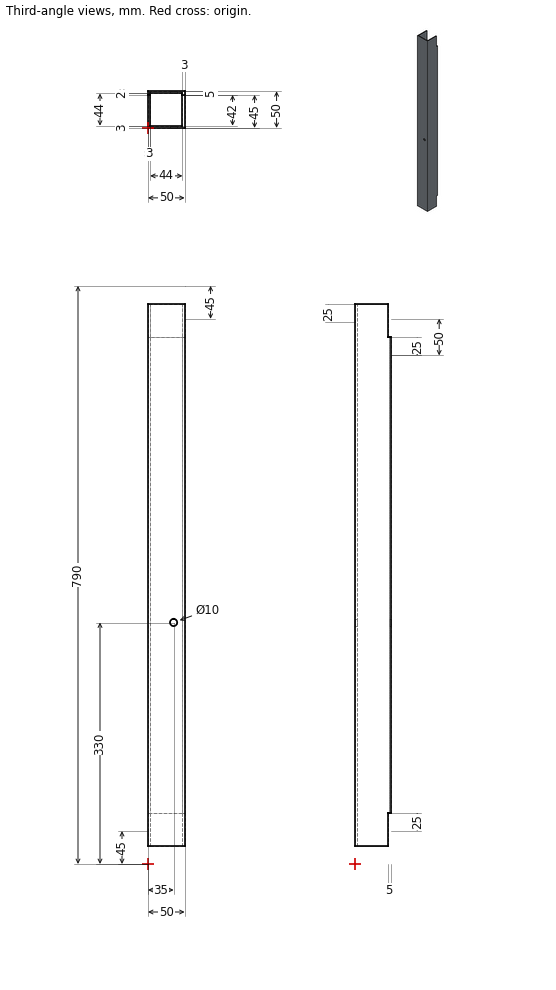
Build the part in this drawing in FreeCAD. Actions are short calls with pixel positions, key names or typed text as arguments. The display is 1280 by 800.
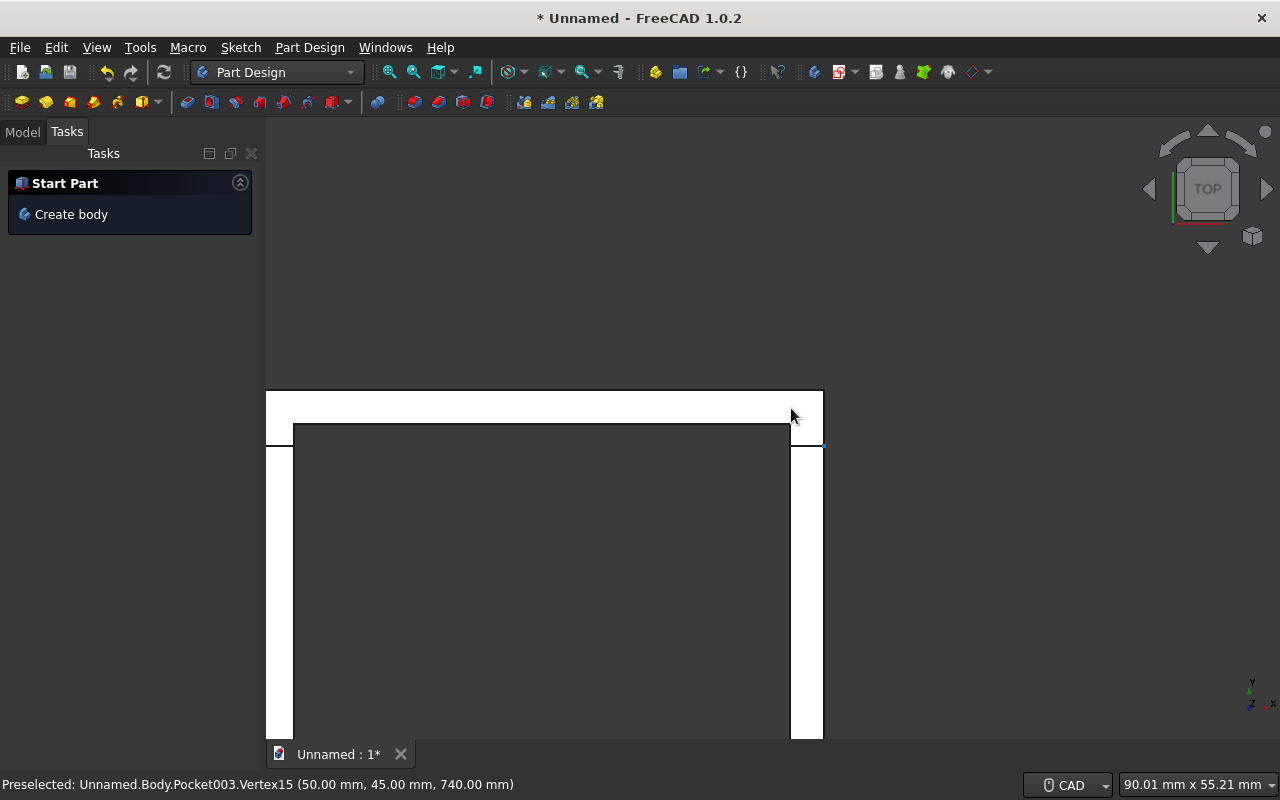
click(784, 409)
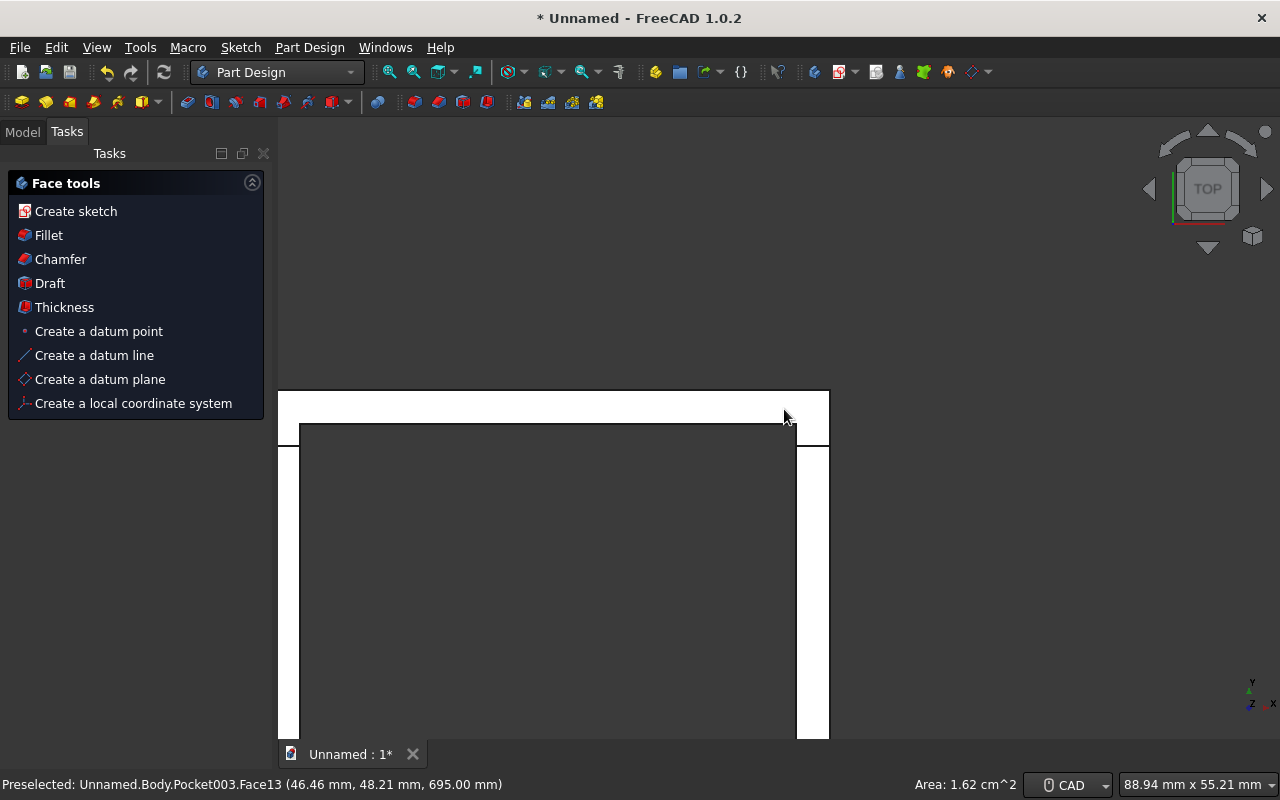
click(840, 72)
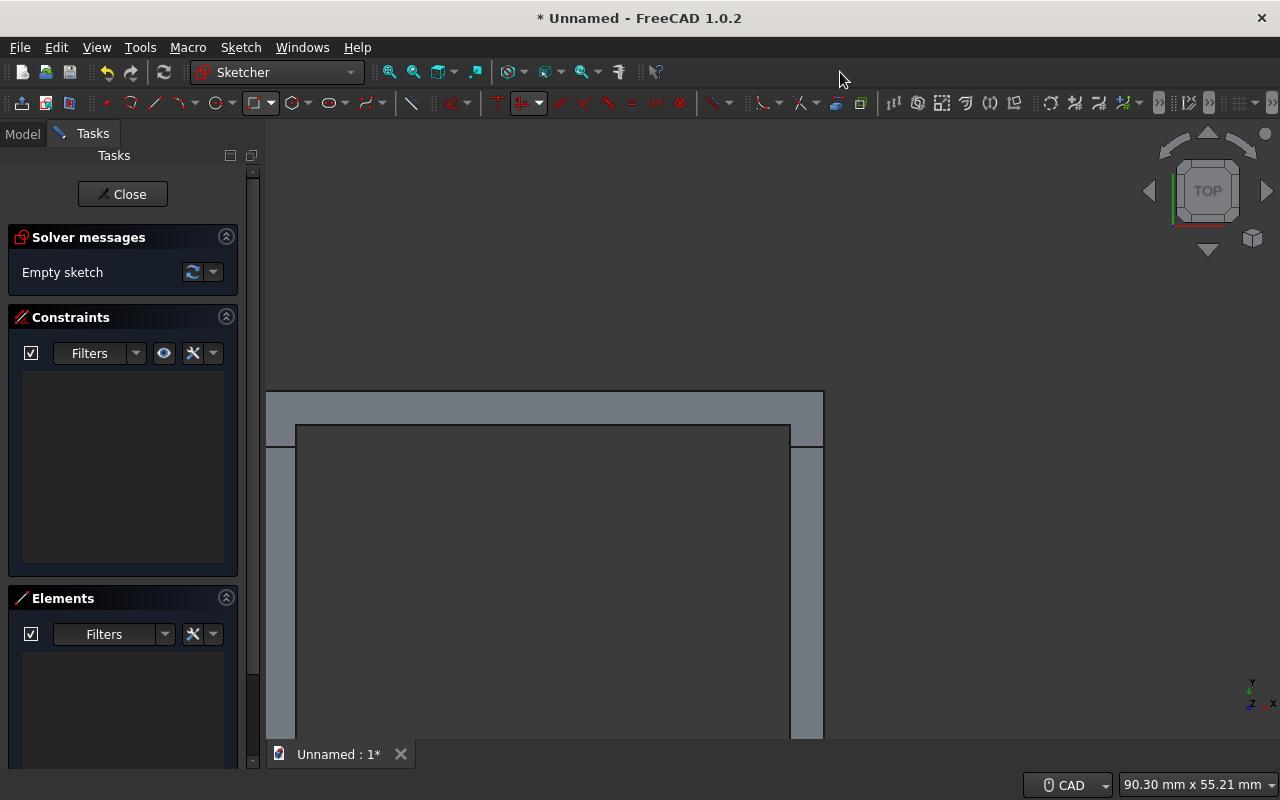
key(q)
key(s)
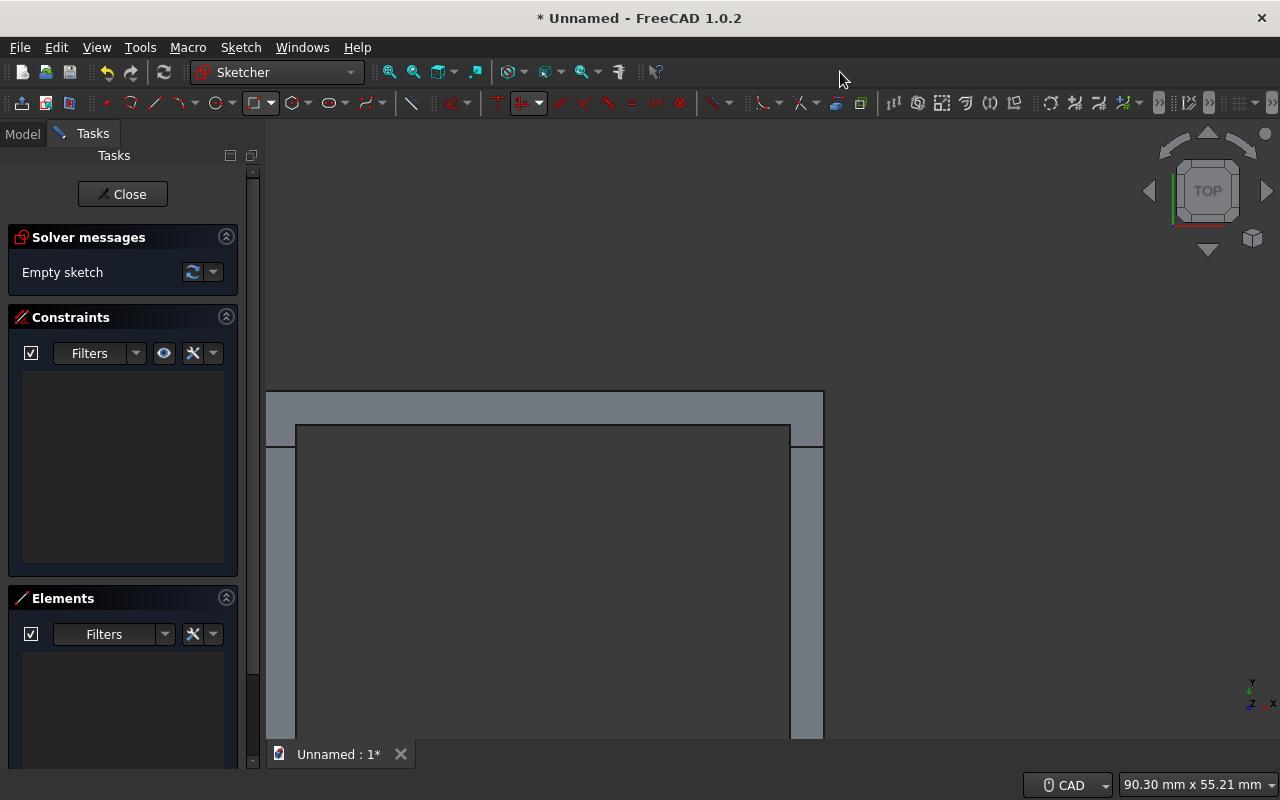
scroll(901, 147, down, 3)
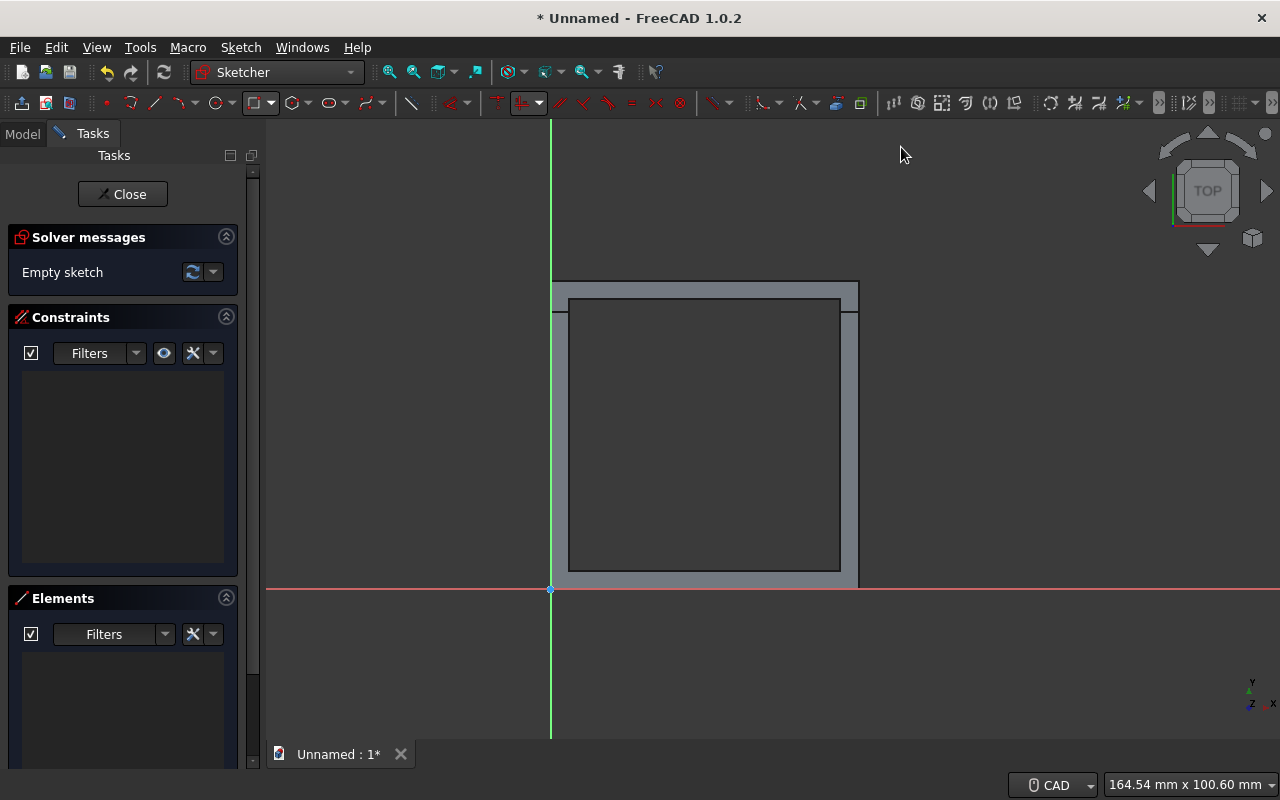
click(132, 104)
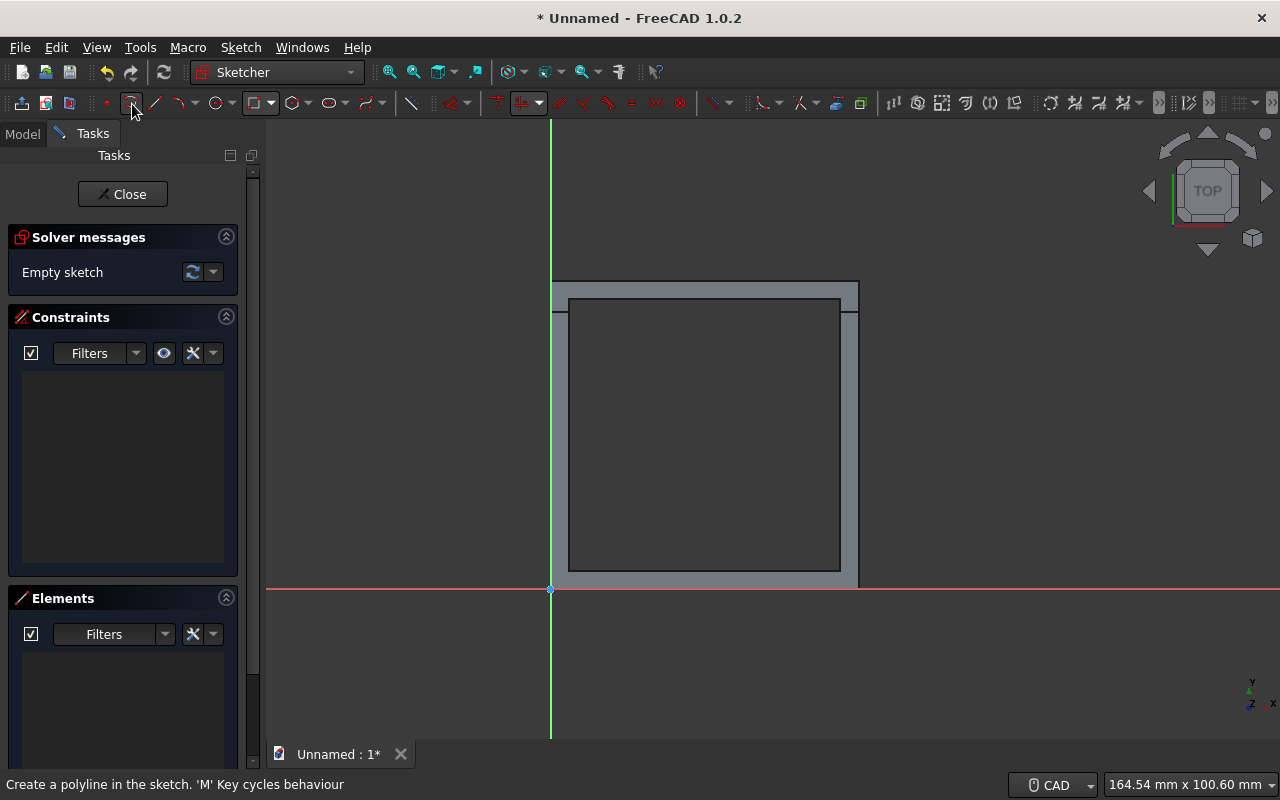
click(551, 312)
click(569, 312)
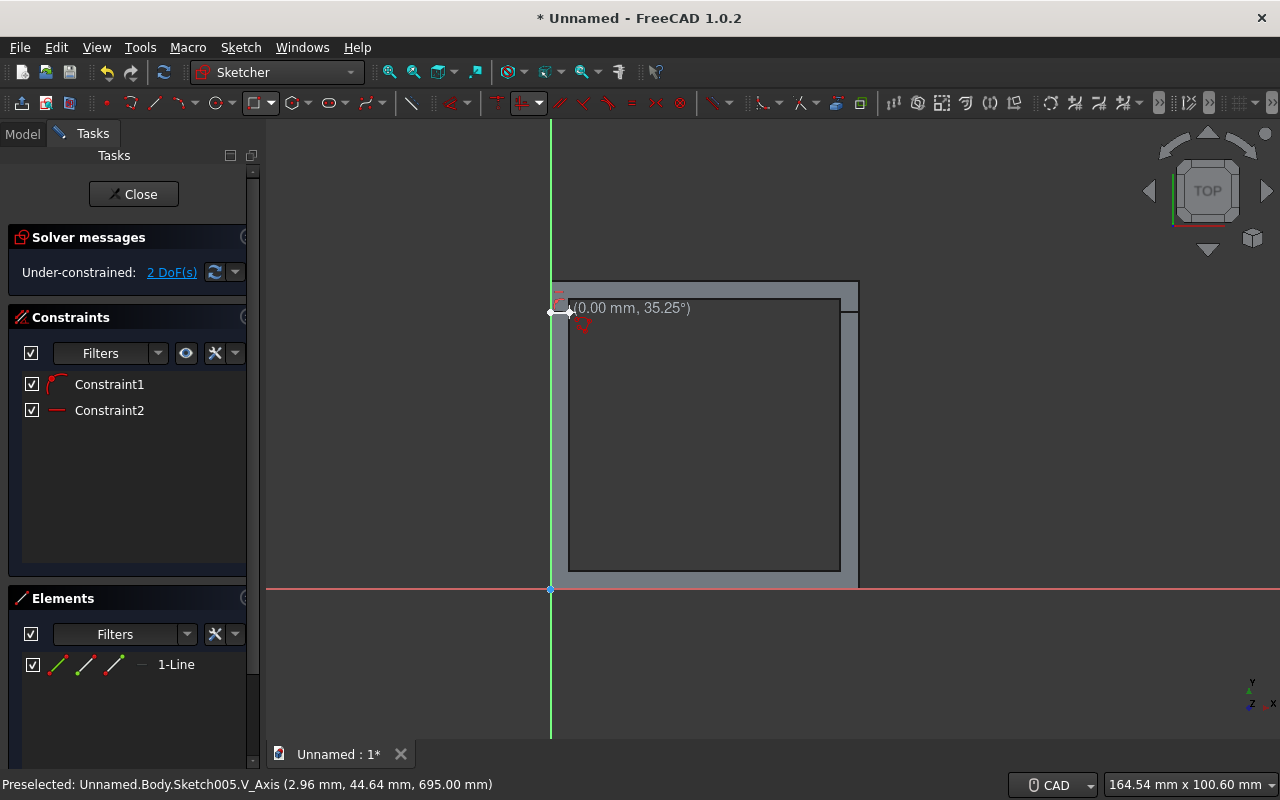
scroll(569, 299, up, 2)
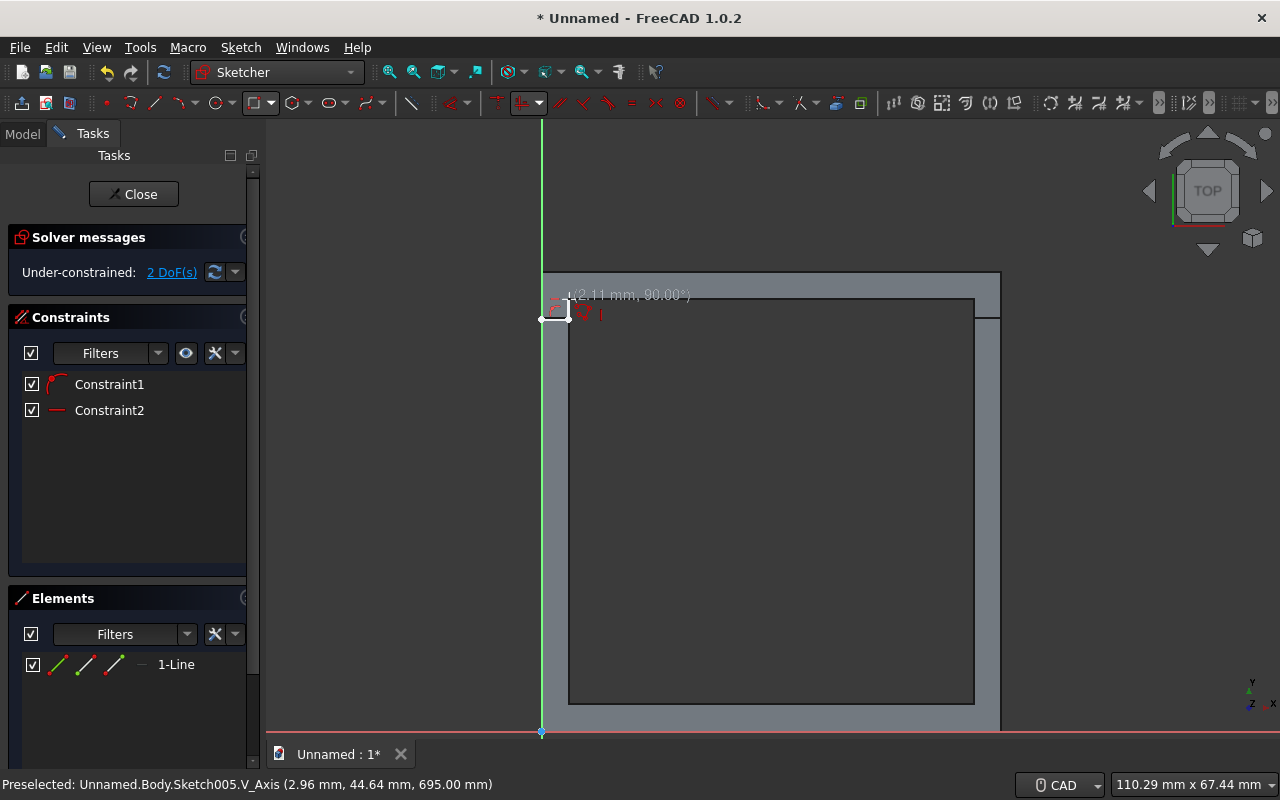
click(569, 299)
click(974, 299)
click(974, 318)
click(1001, 318)
click(1001, 272)
click(551, 272)
click(542, 320)
key(Escape)
key(Escape)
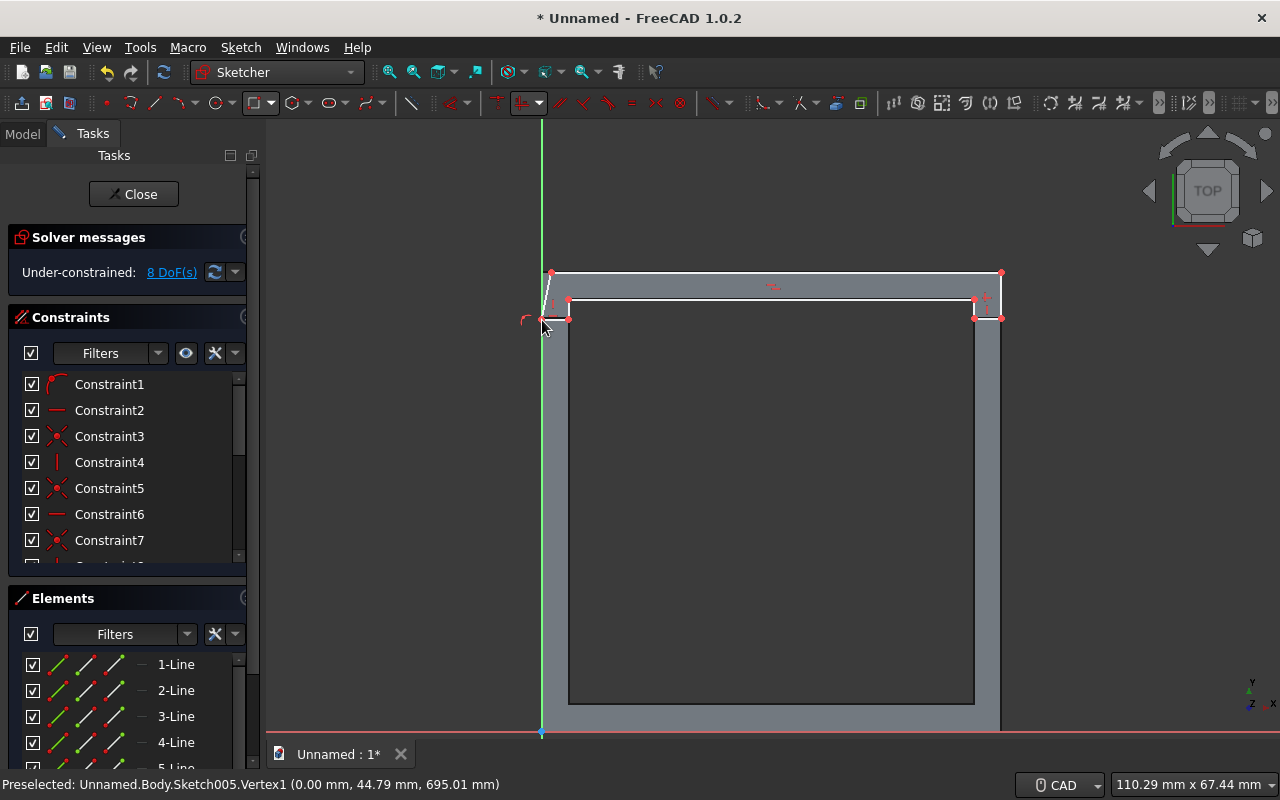
click(544, 306)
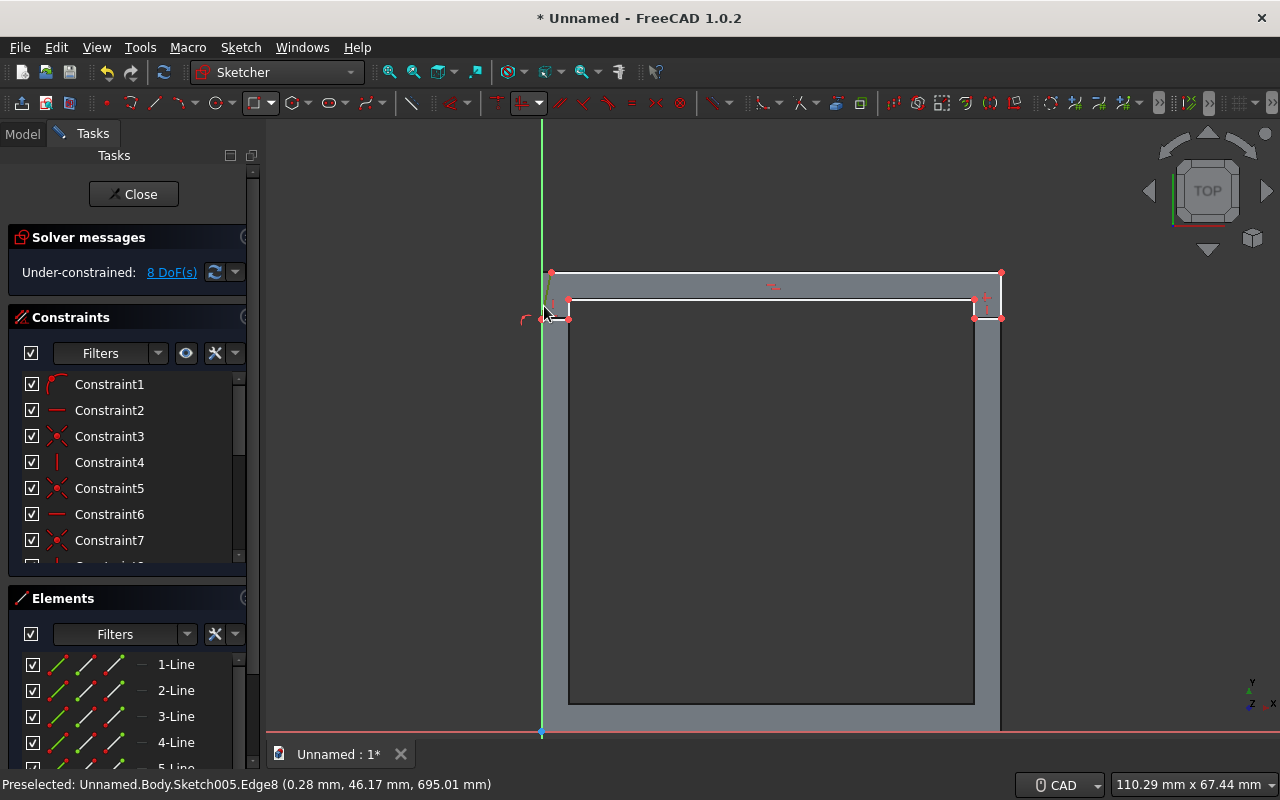
click(542, 104)